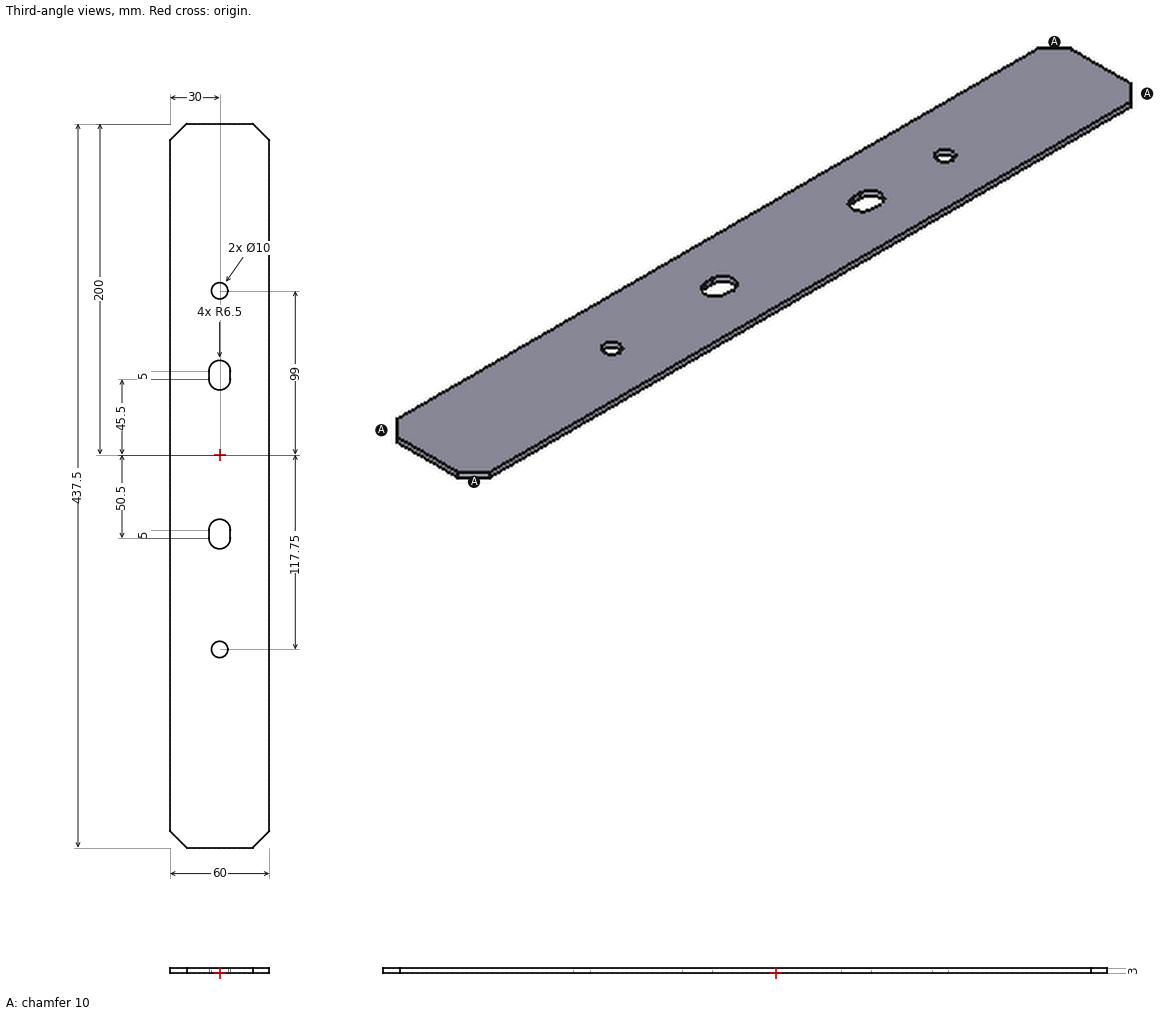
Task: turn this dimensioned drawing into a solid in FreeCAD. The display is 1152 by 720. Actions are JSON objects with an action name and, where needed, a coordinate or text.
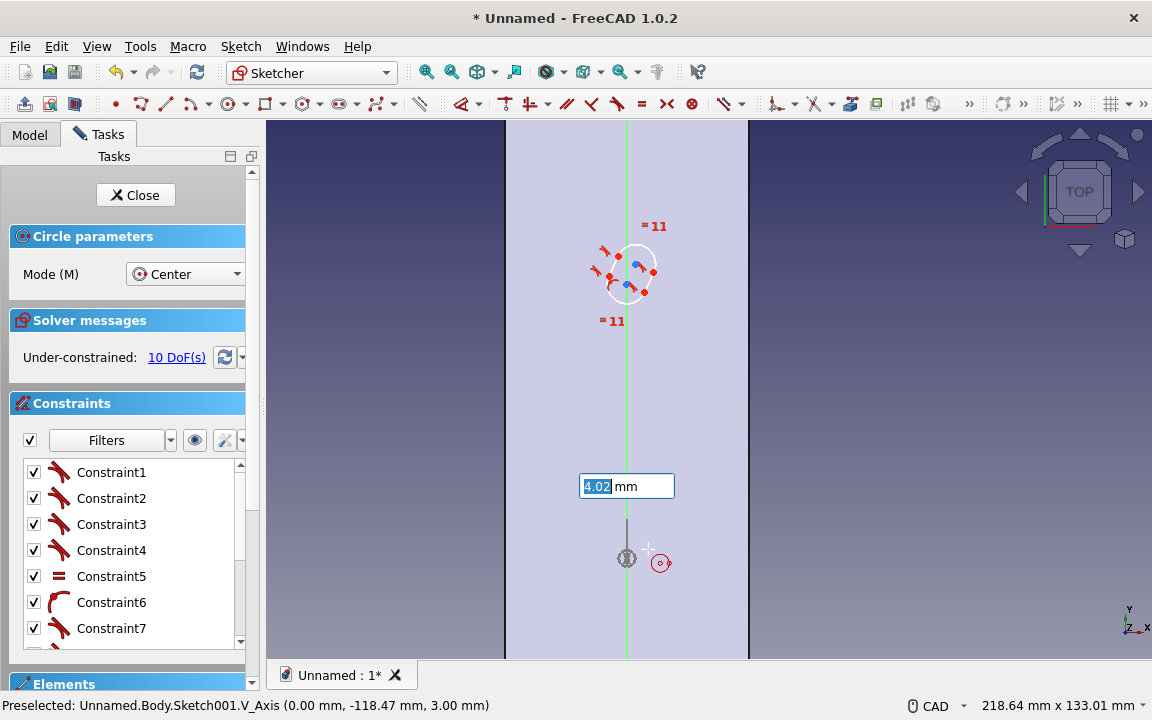
{"action": "left_click", "coordinate": [646, 549]}
{"action": "key", "text": "Escape"}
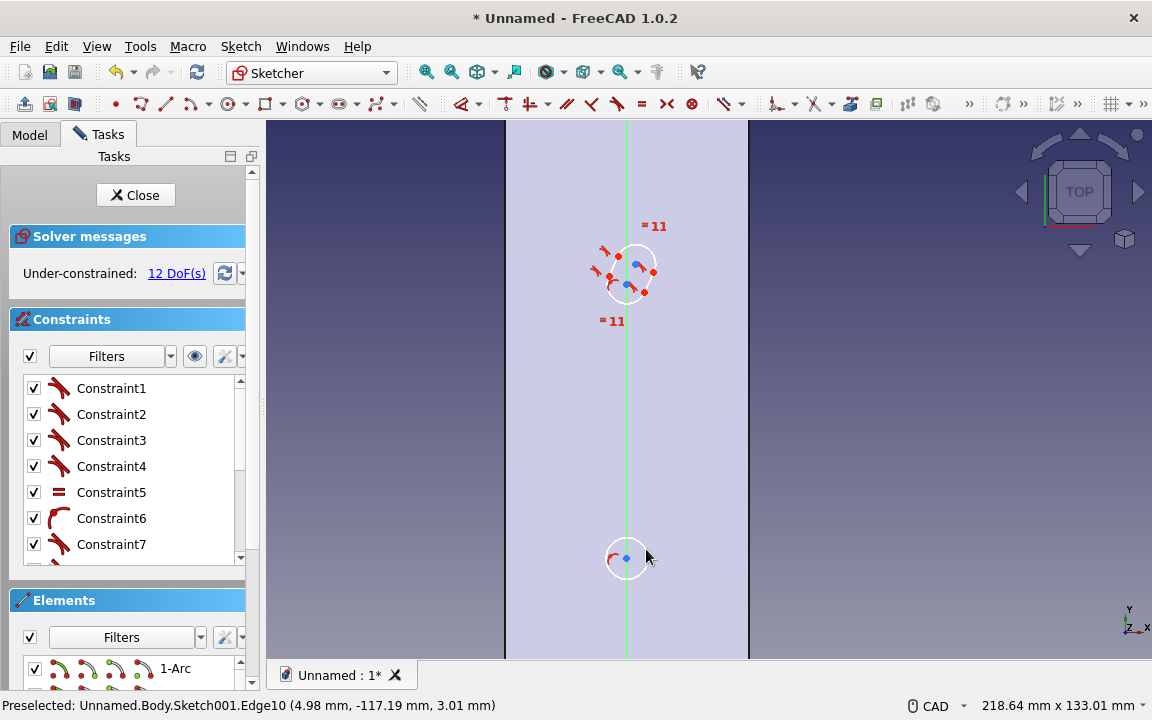
{"action": "scroll", "coordinate": [648, 548], "scroll_direction": "down", "scroll_amount": 5}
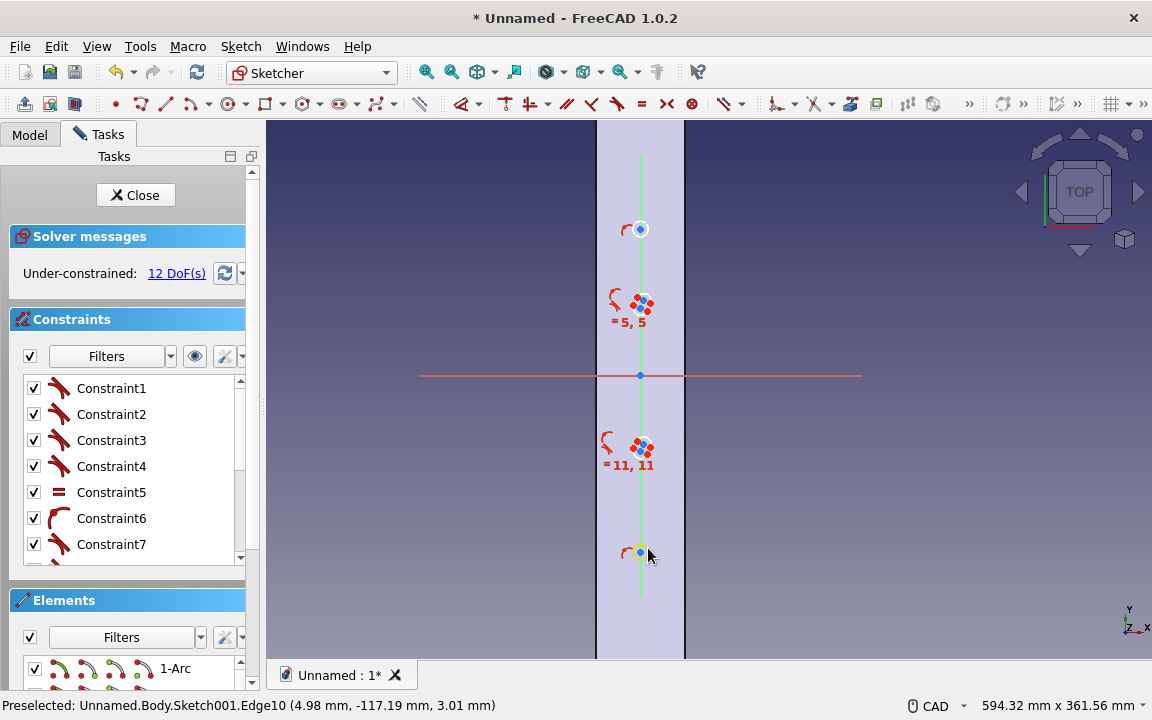
{"action": "scroll", "coordinate": [636, 301], "scroll_direction": "up", "scroll_amount": 7}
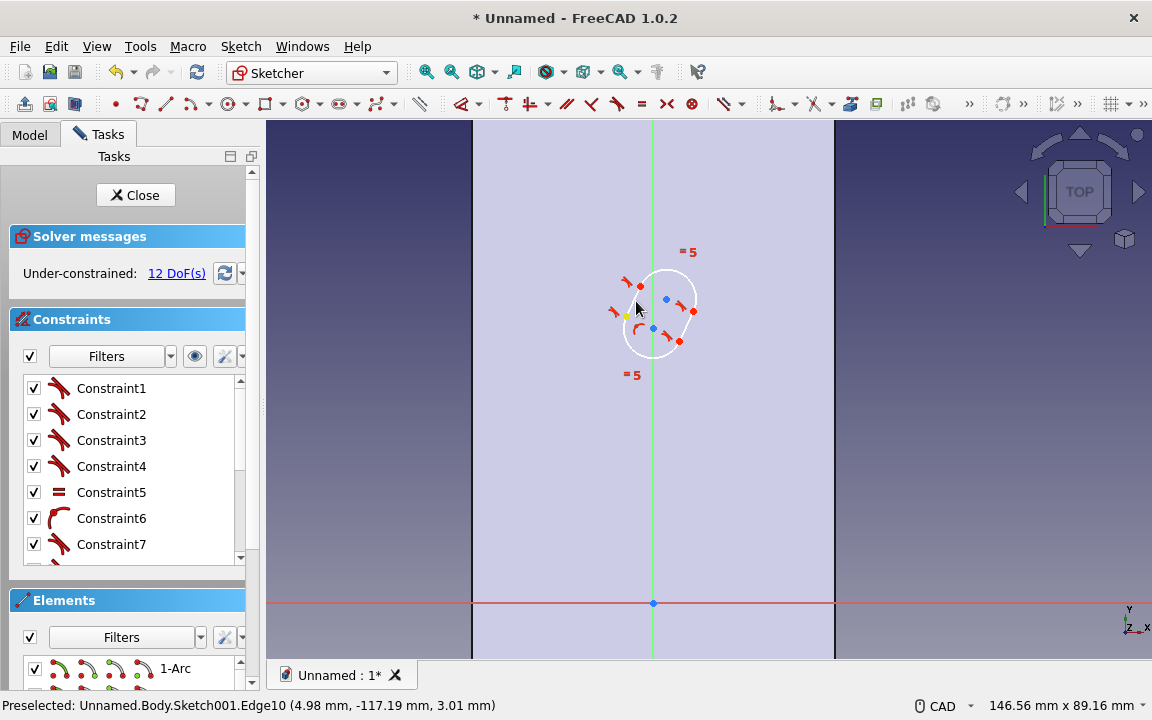
{"action": "left_click", "coordinate": [633, 302]}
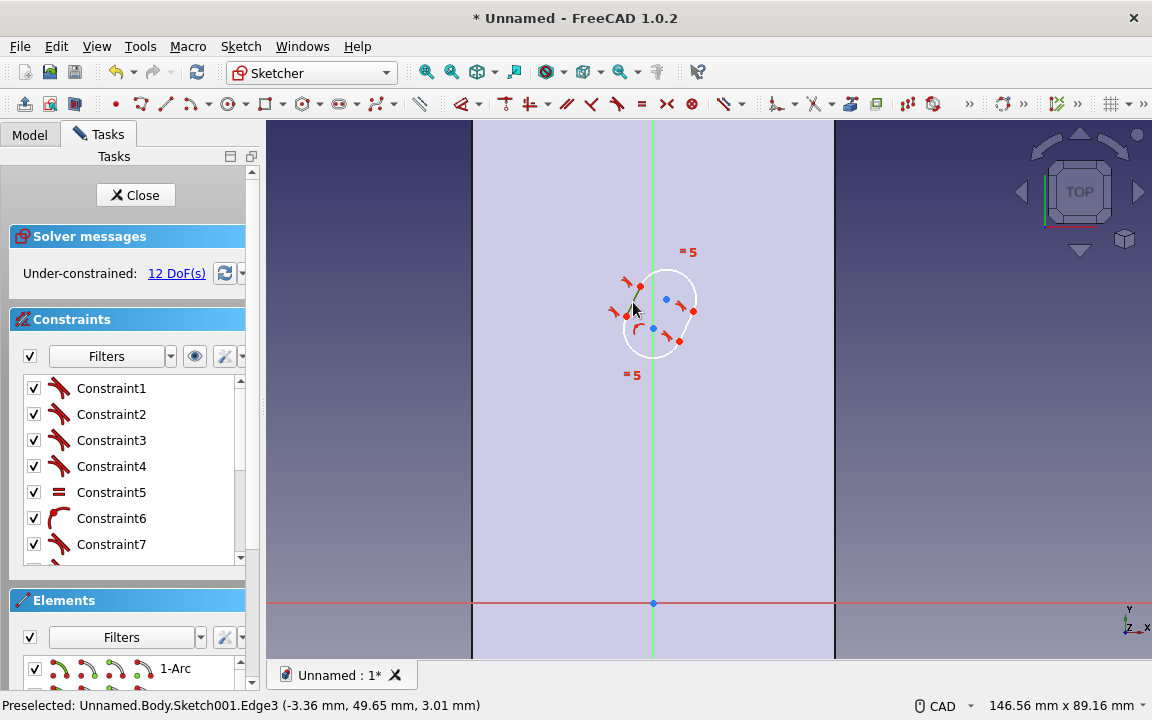
{"action": "left_click", "coordinate": [548, 104]}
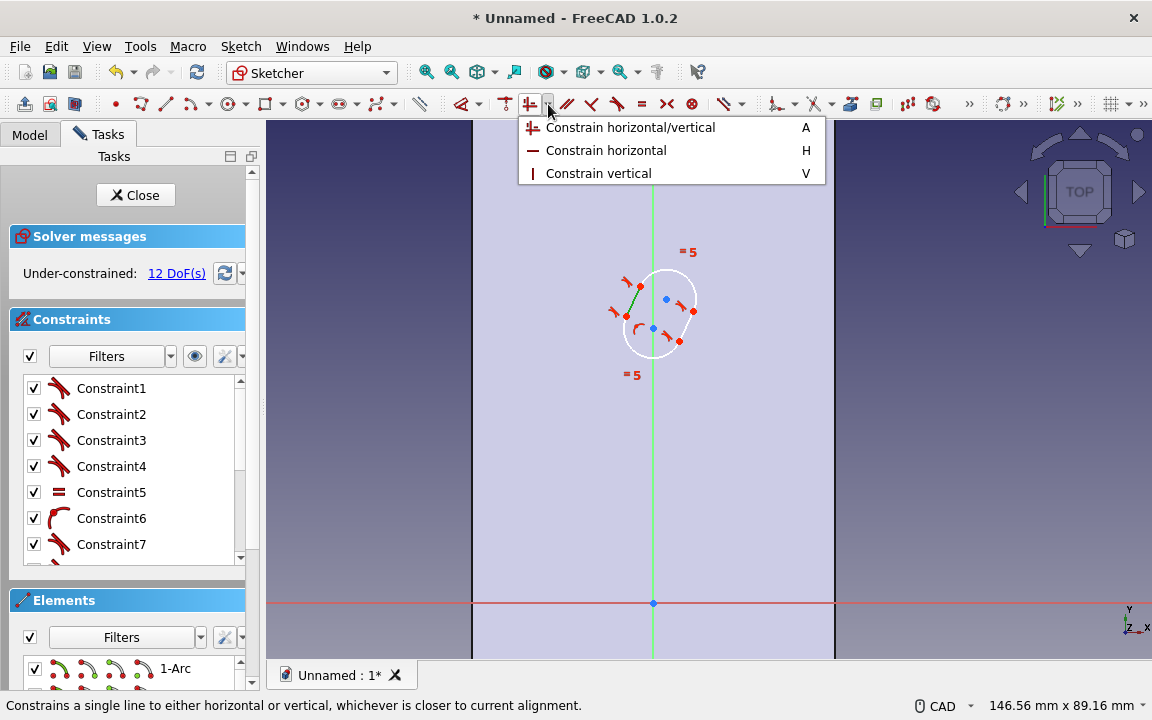
{"action": "left_click", "coordinate": [672, 174]}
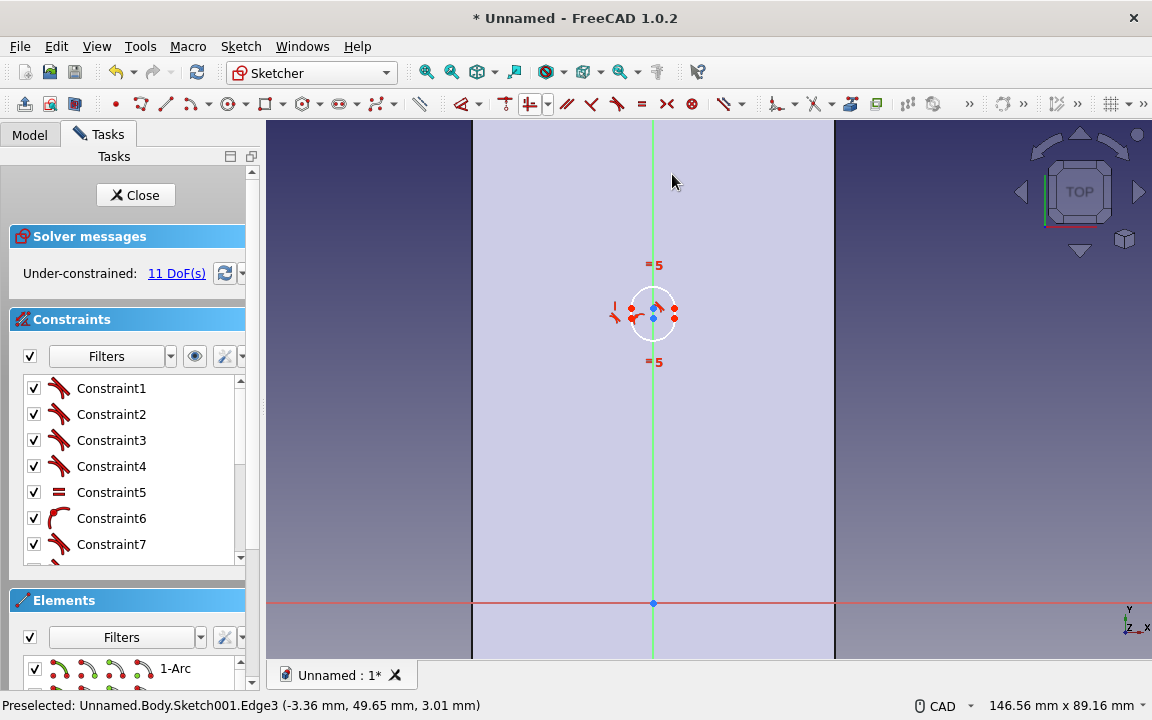
{"action": "scroll", "coordinate": [636, 301], "scroll_direction": "down", "scroll_amount": 7}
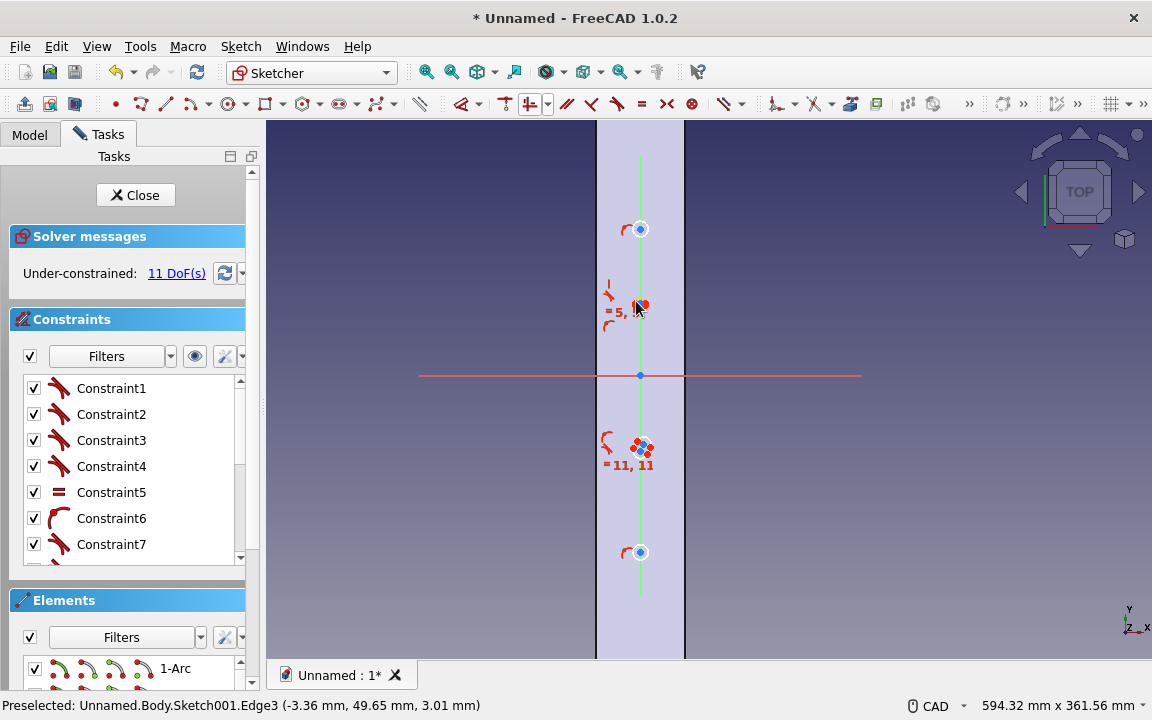
{"action": "scroll", "coordinate": [635, 446], "scroll_direction": "up", "scroll_amount": 9}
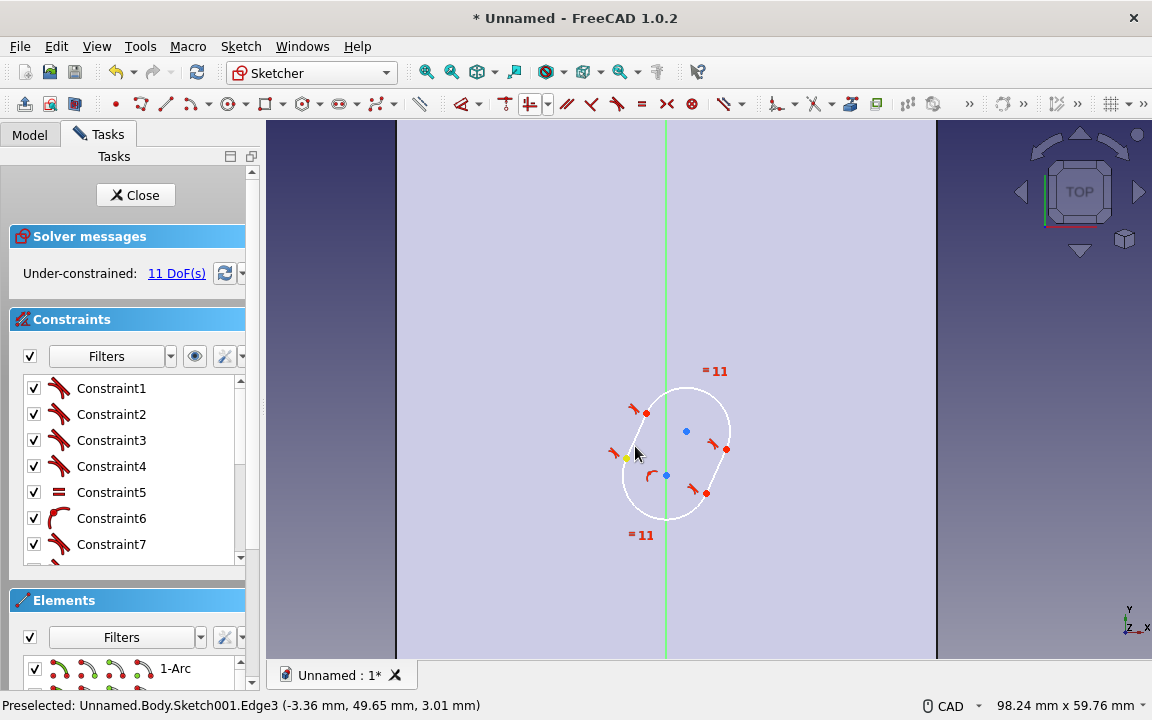
{"action": "left_click", "coordinate": [633, 445]}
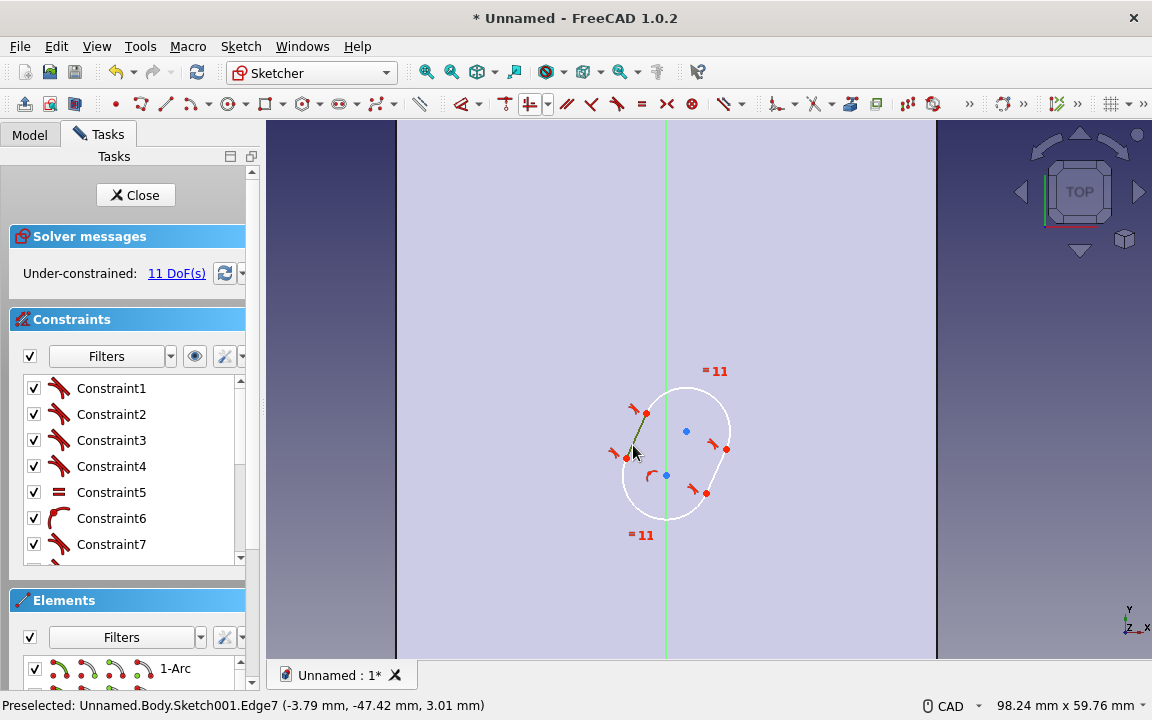
{"action": "left_click", "coordinate": [548, 104]}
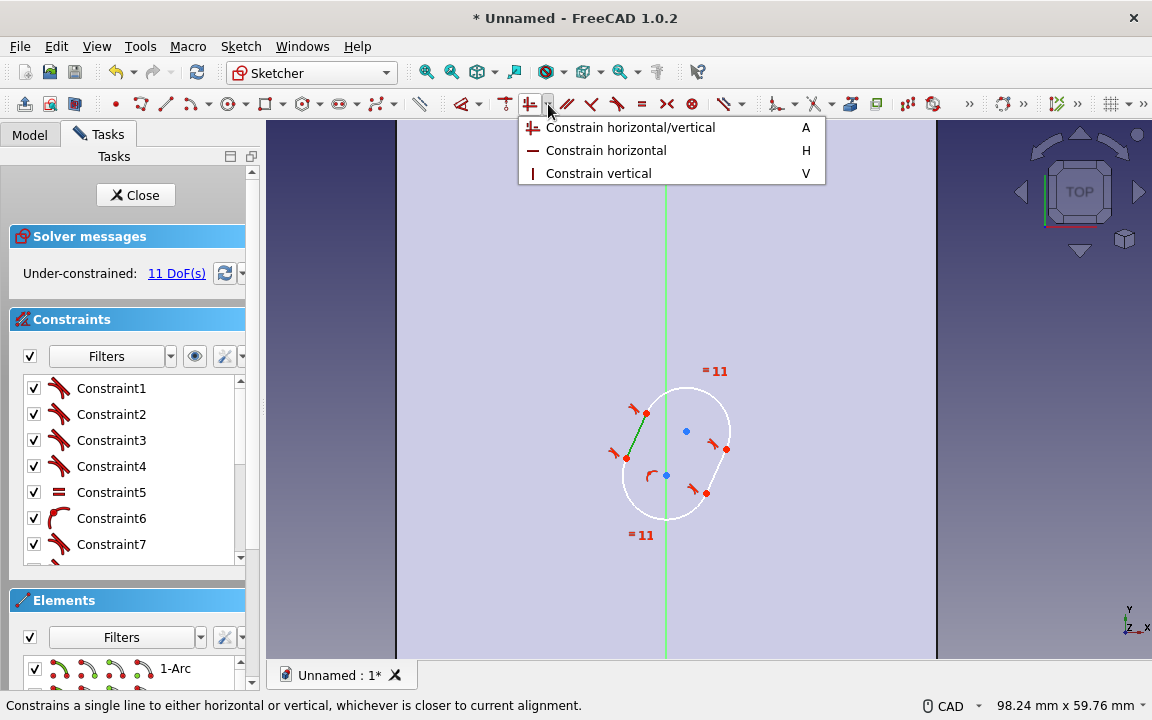
{"action": "left_click", "coordinate": [672, 174]}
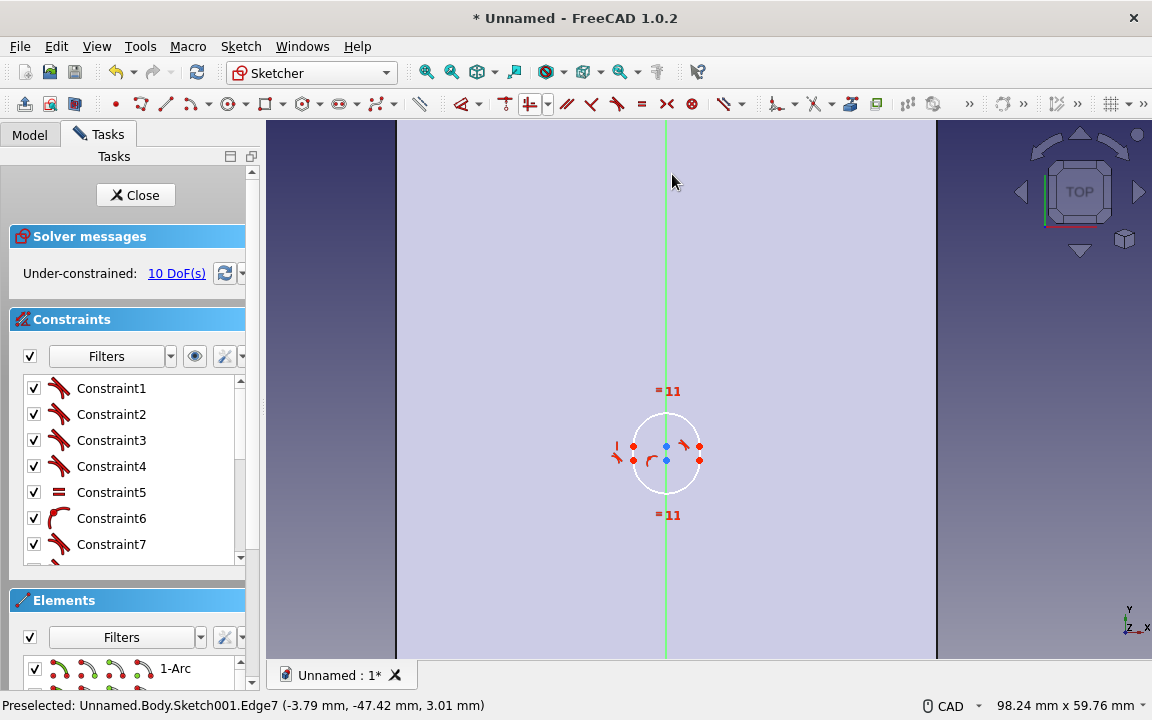
{"action": "scroll", "coordinate": [635, 446], "scroll_direction": "down", "scroll_amount": 9}